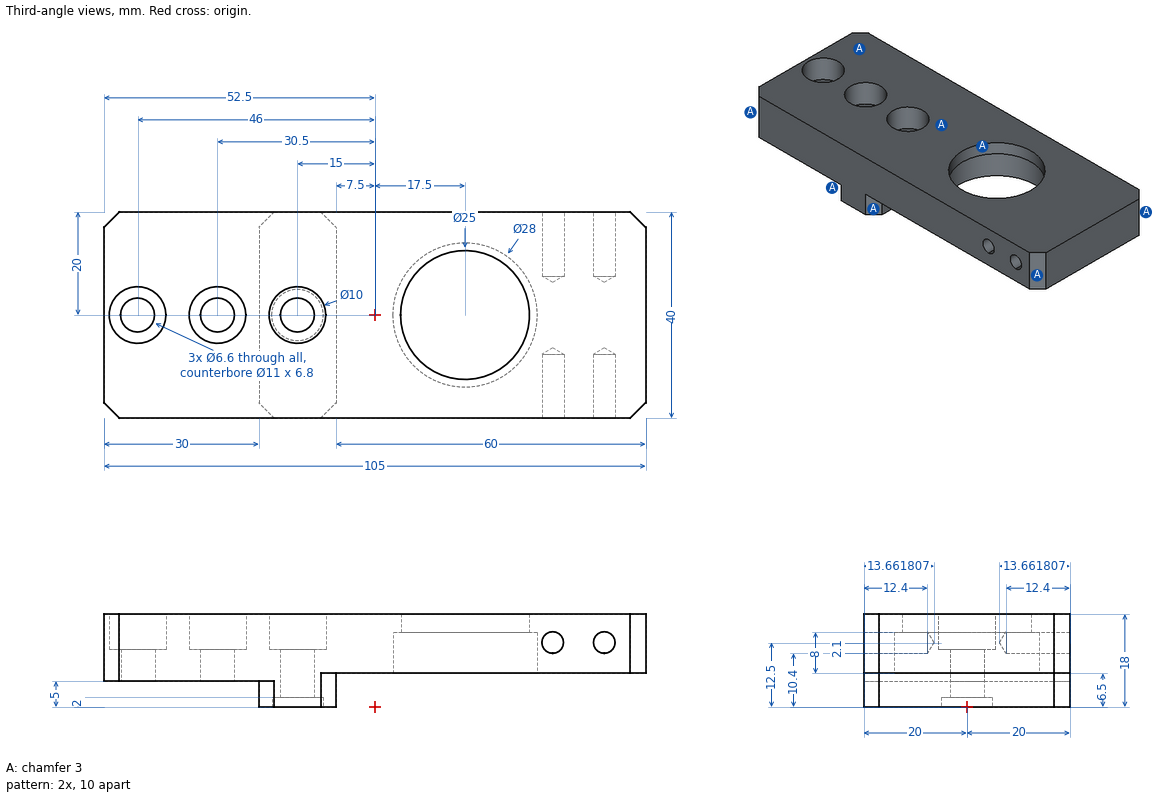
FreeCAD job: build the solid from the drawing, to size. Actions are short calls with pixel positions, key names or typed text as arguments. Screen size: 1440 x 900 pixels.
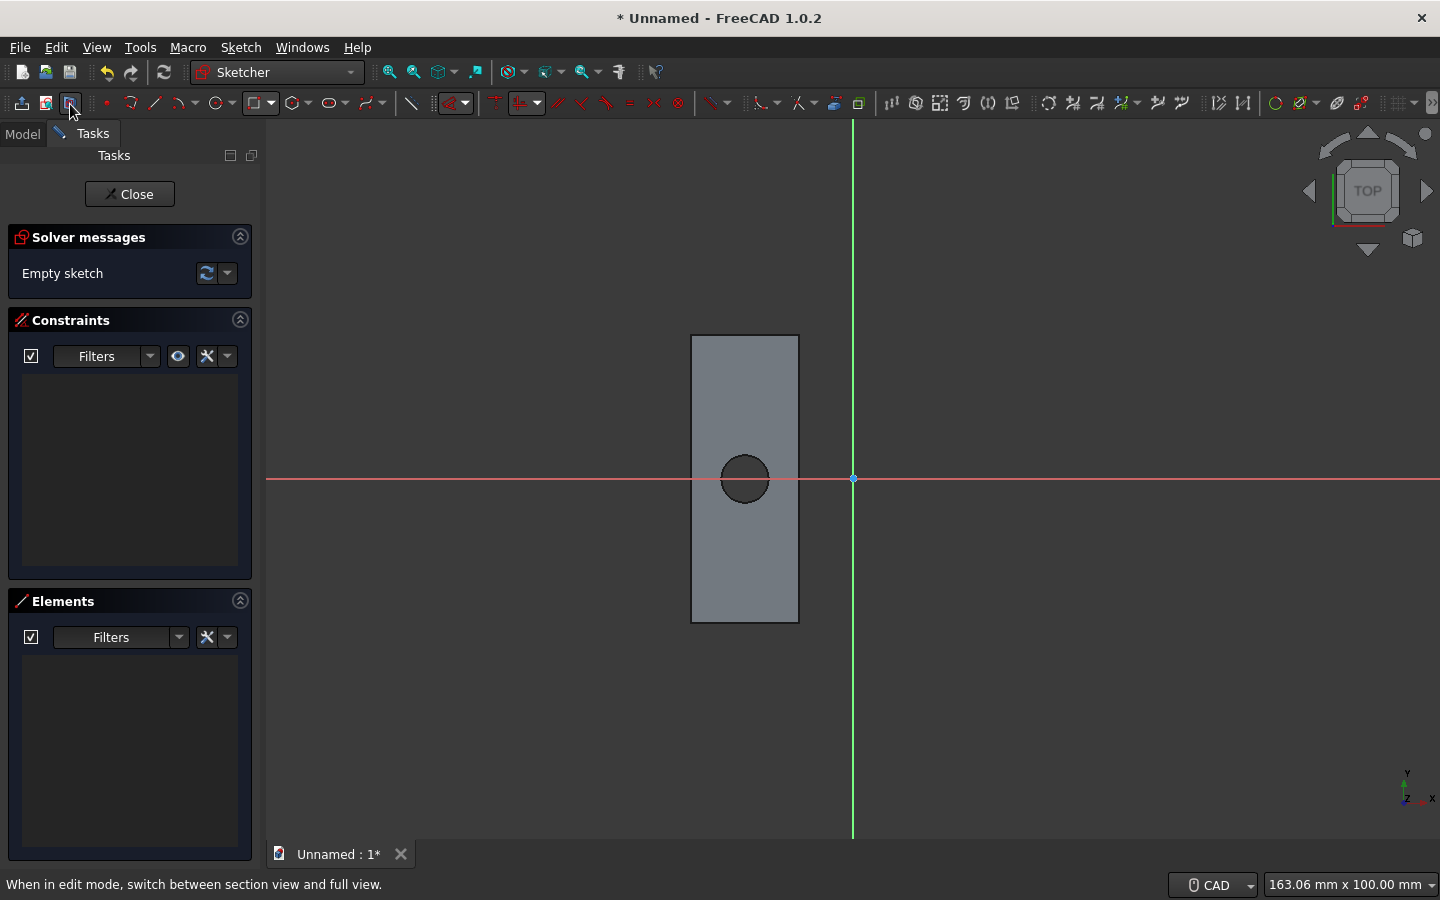
scroll(780, 479, up, 8)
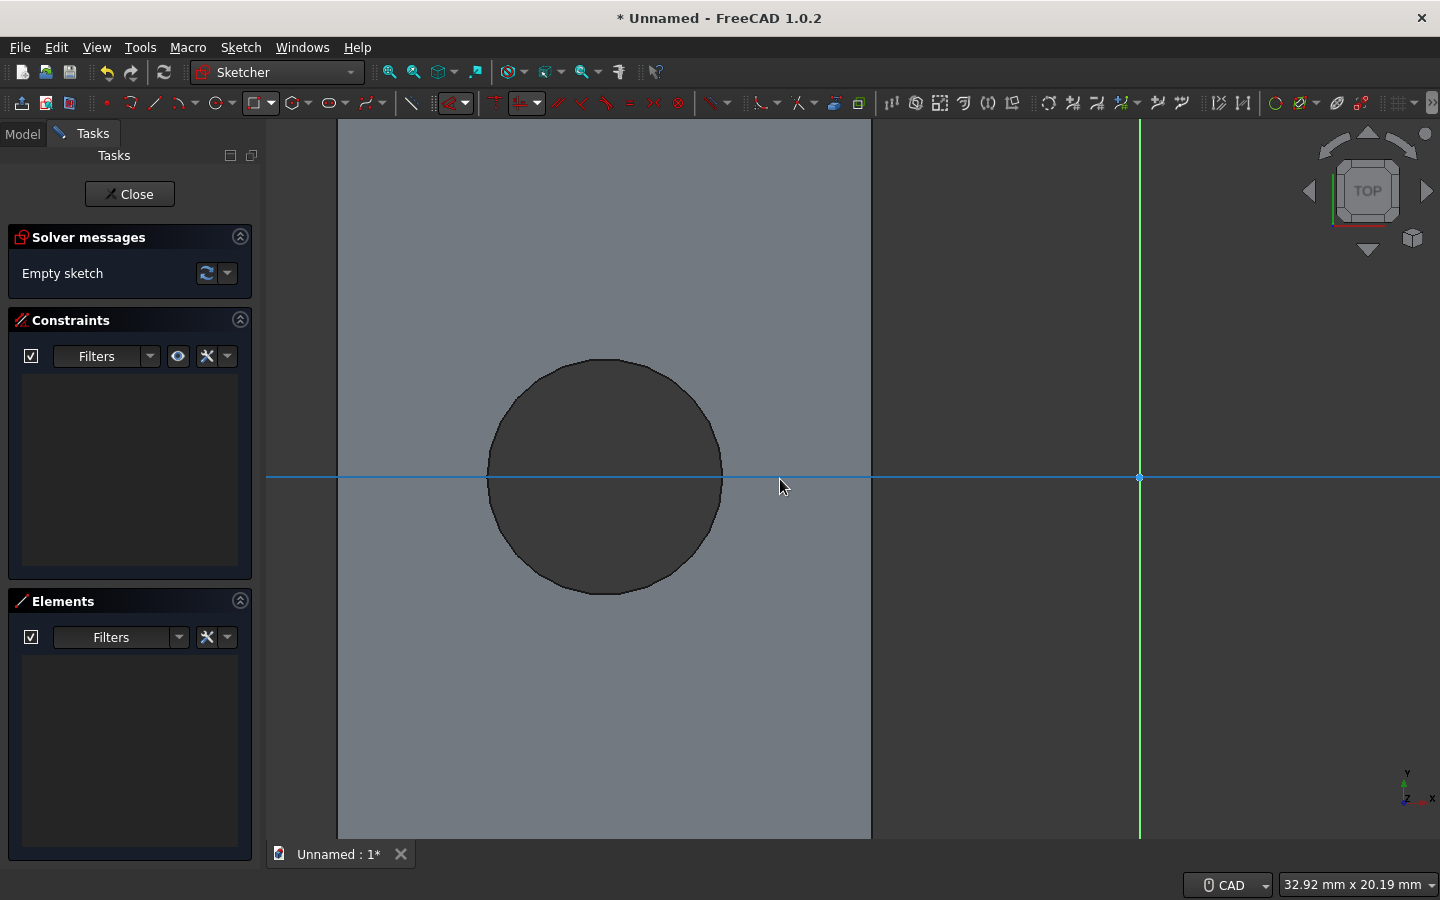
click(216, 104)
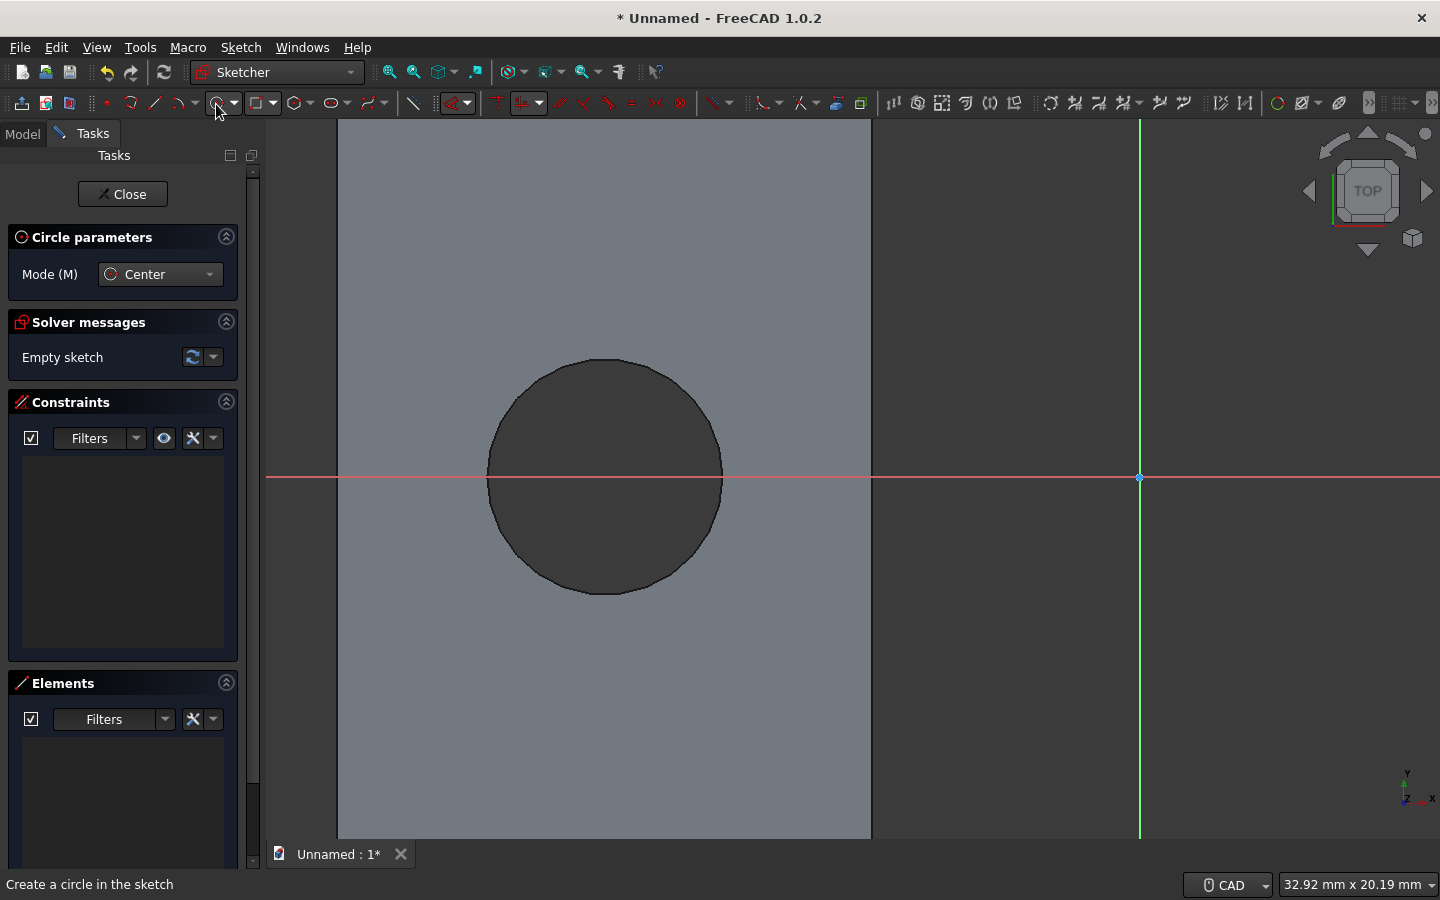
click(605, 477)
click(731, 351)
key(Escape)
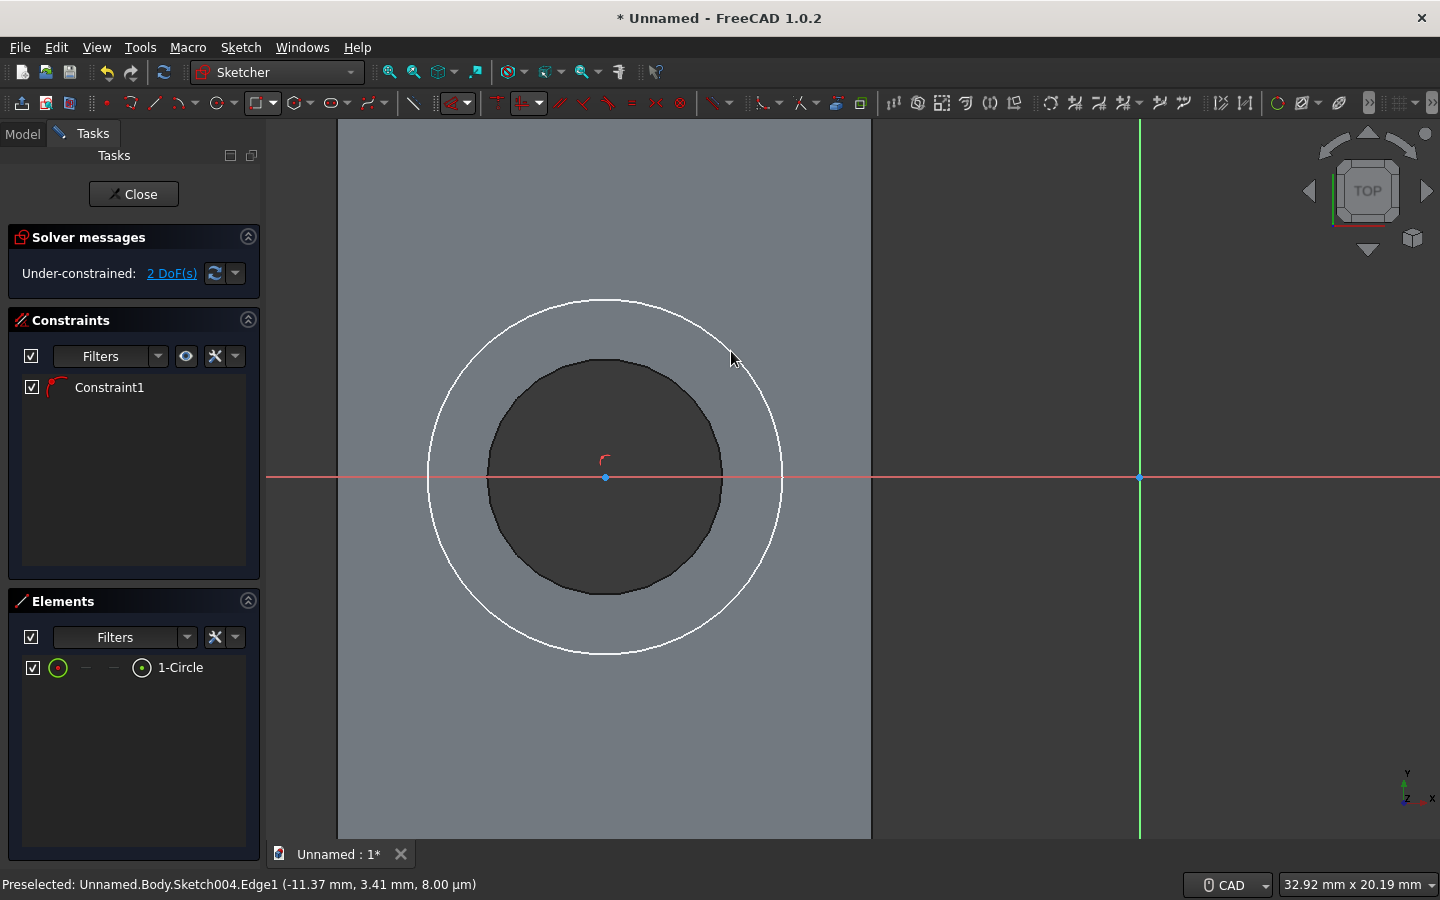
click(730, 351)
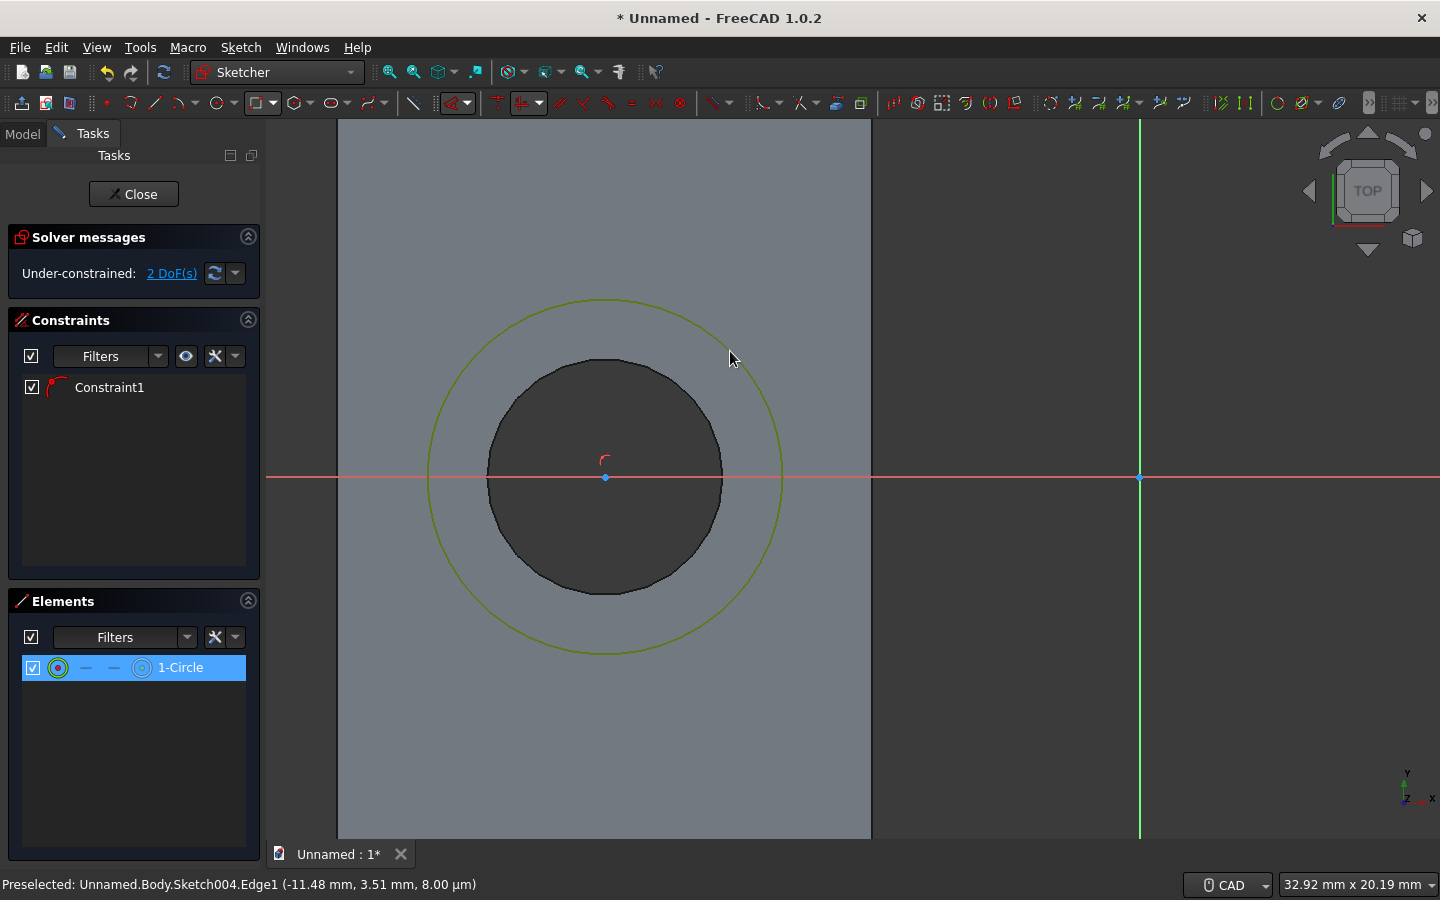
click(470, 104)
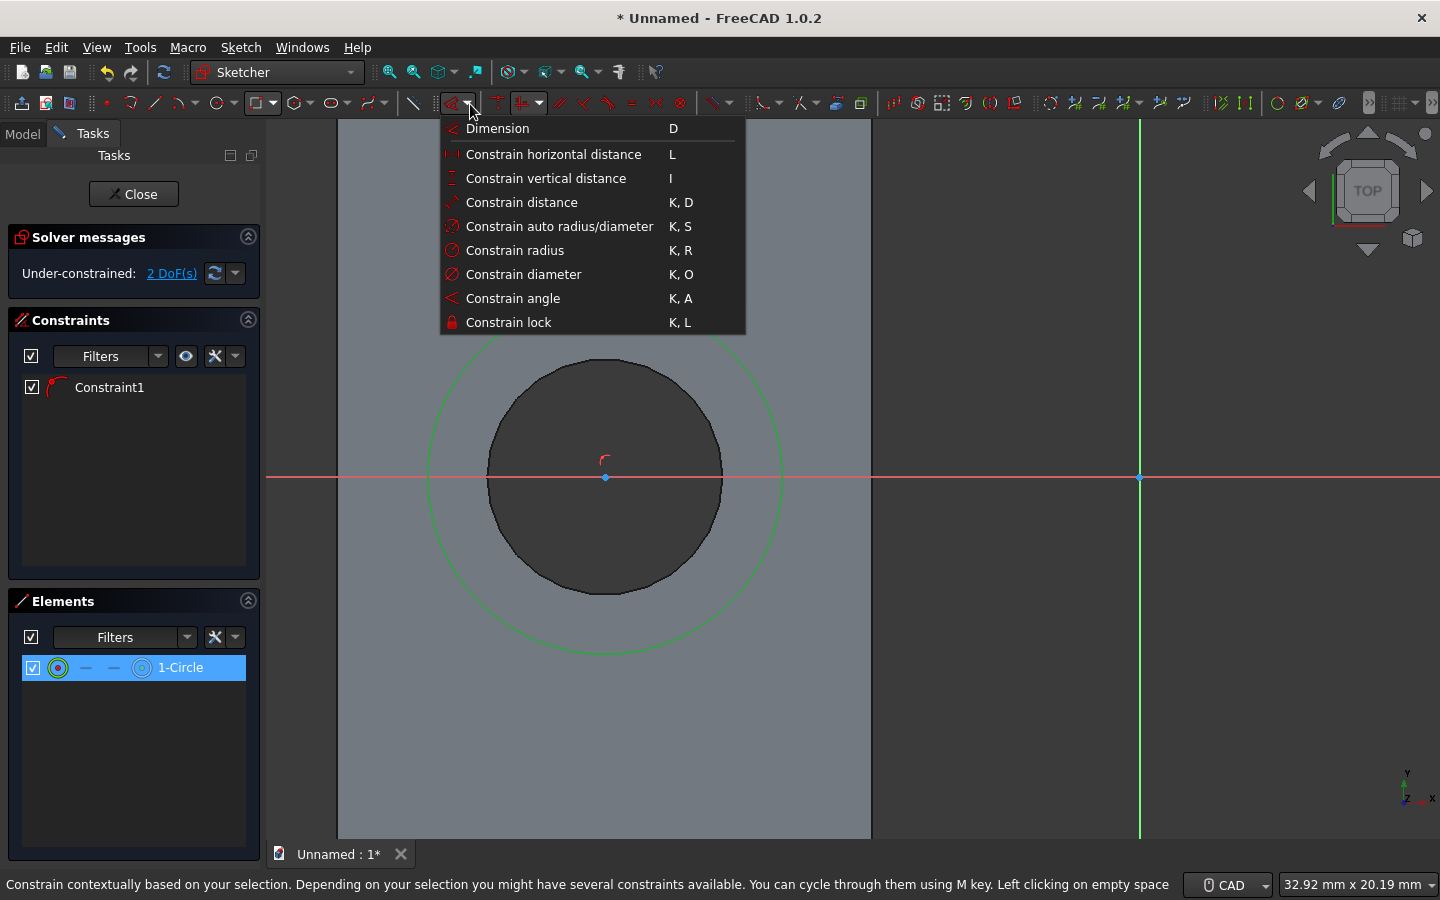
click(593, 274)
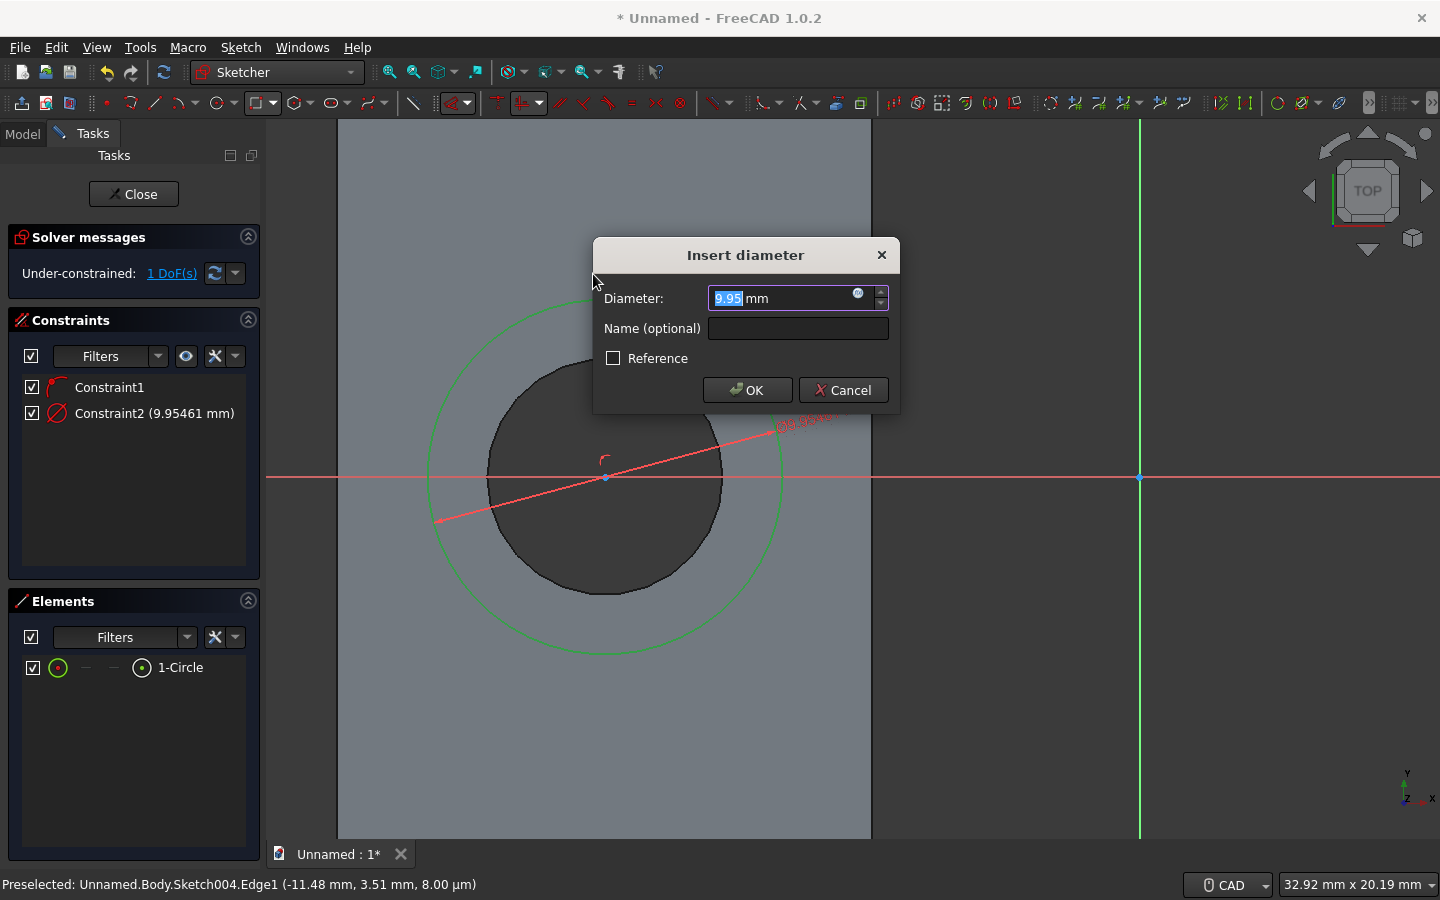
text(10)
key(Return)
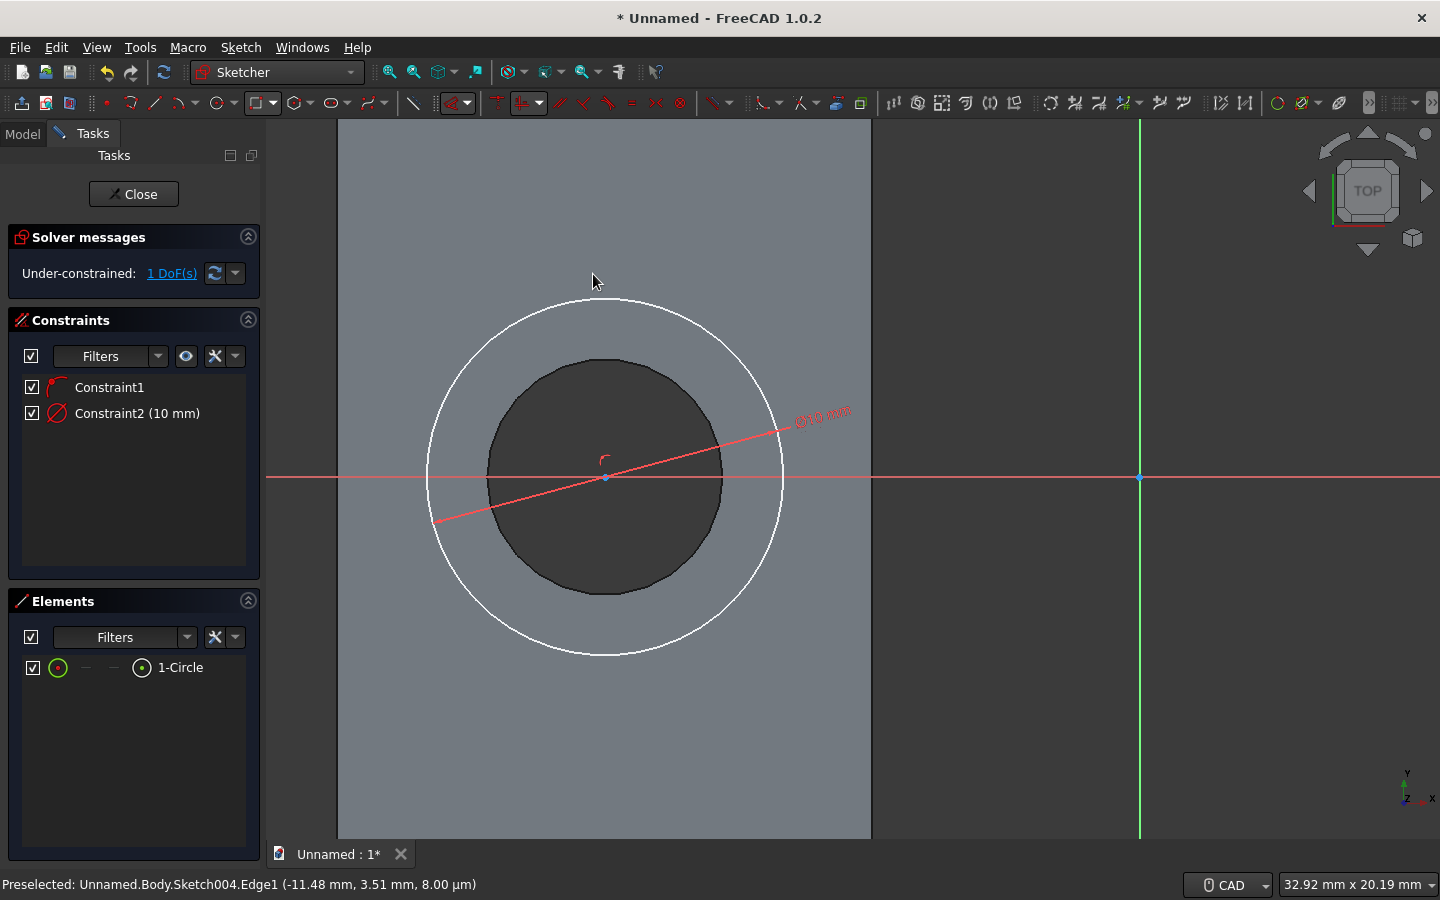
click(605, 477)